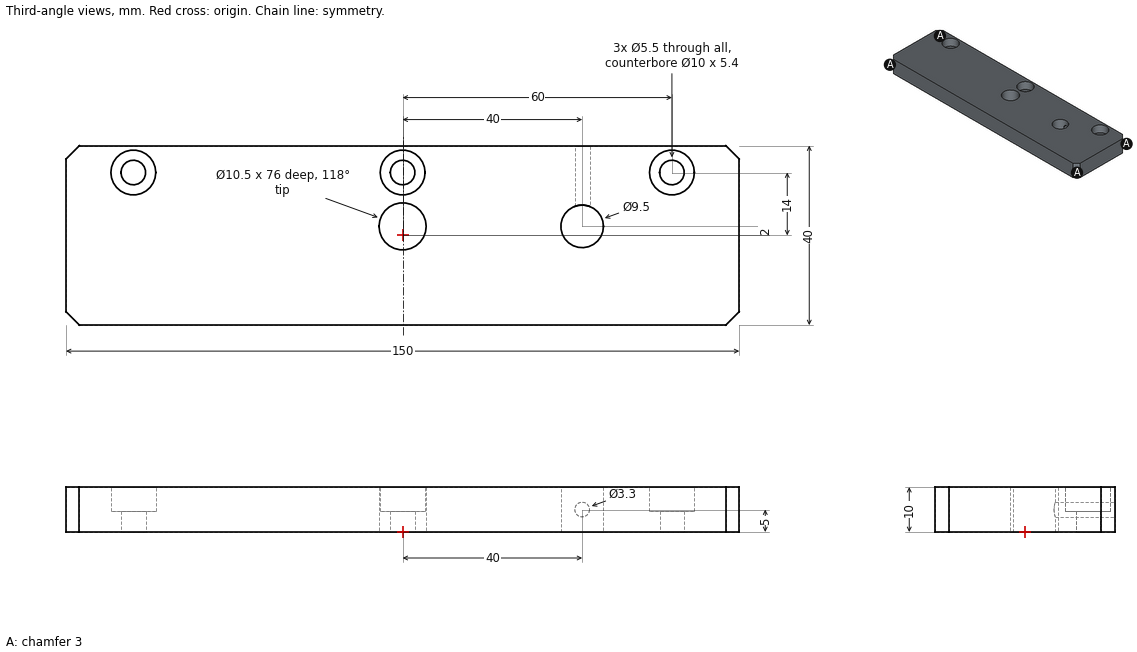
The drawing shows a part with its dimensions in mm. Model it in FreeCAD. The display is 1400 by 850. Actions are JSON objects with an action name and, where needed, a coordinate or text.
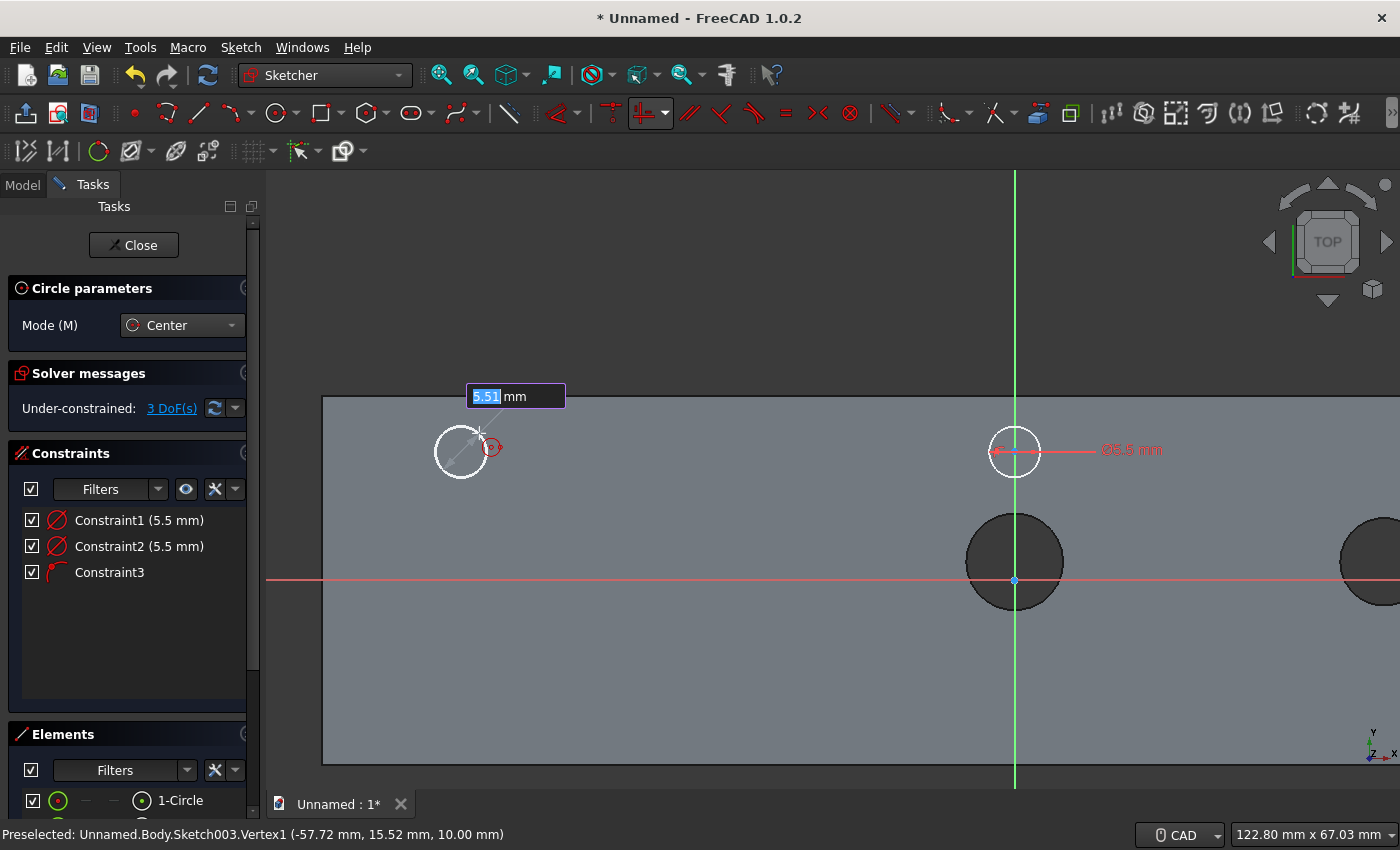
{"action": "type", "text": "5.5"}
{"action": "key", "text": "Return"}
{"action": "key", "text": "Escape"}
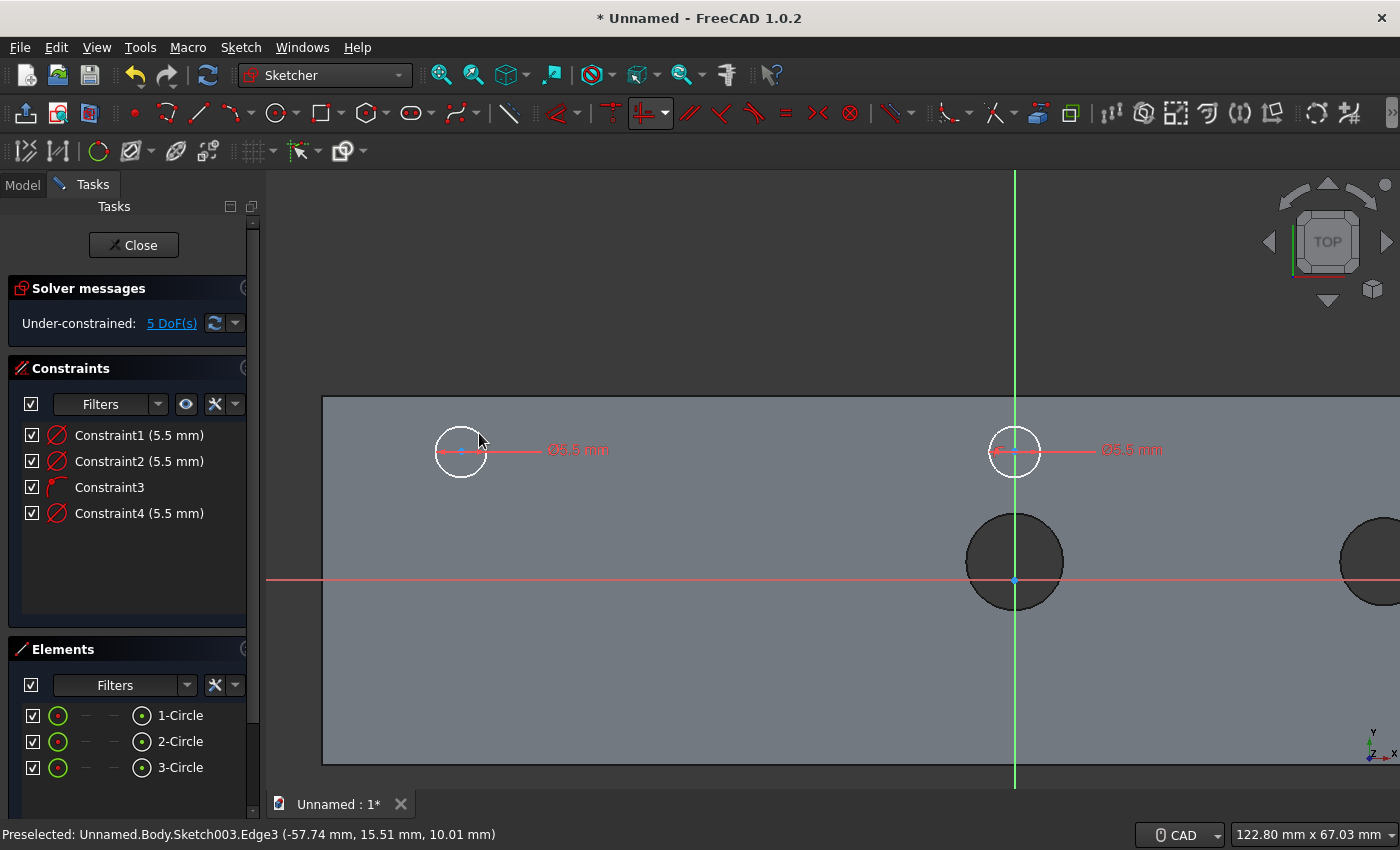
{"action": "scroll", "coordinate": [460, 451], "scroll_direction": "down", "scroll_amount": 3}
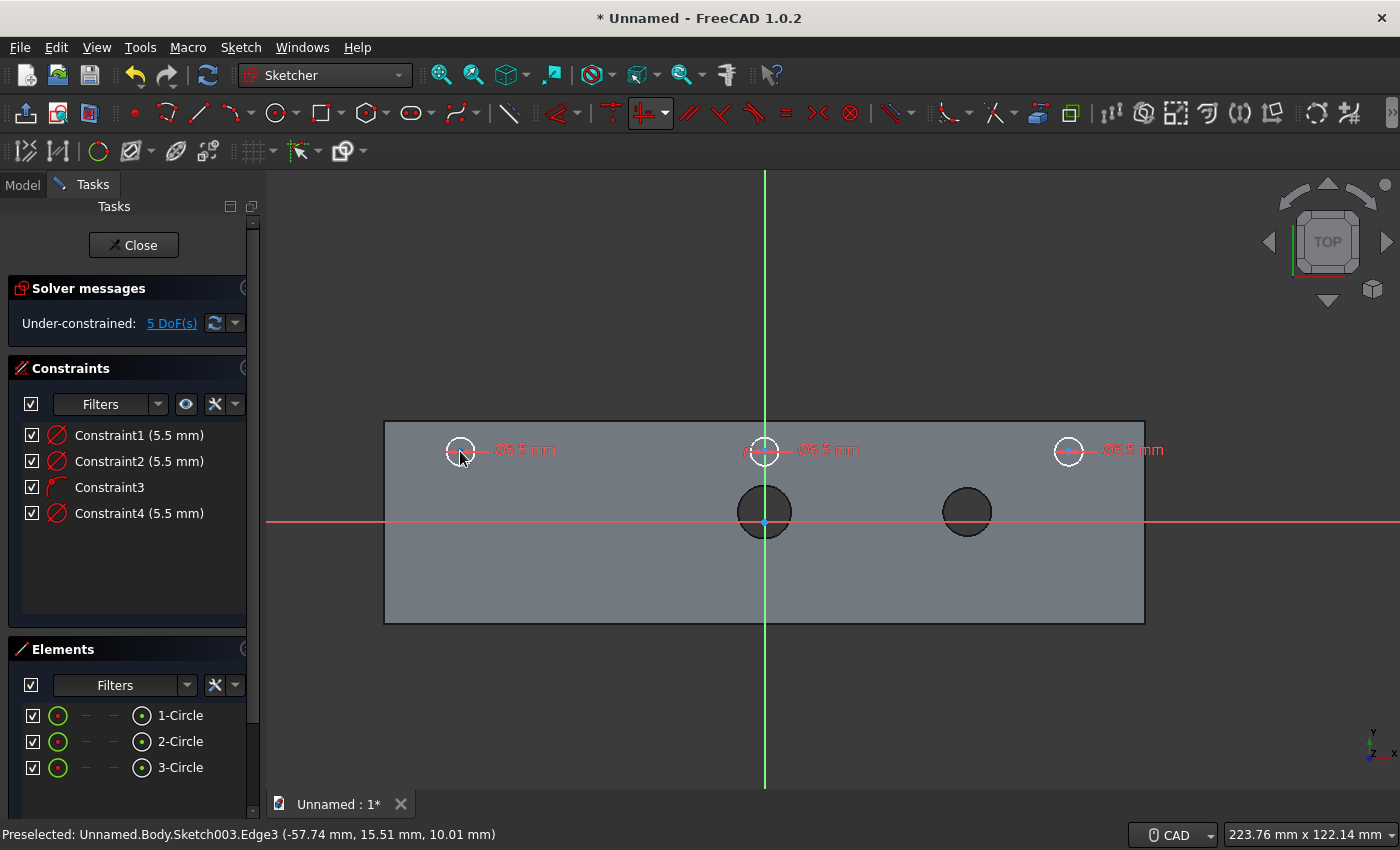
{"action": "left_click", "coordinate": [1069, 452]}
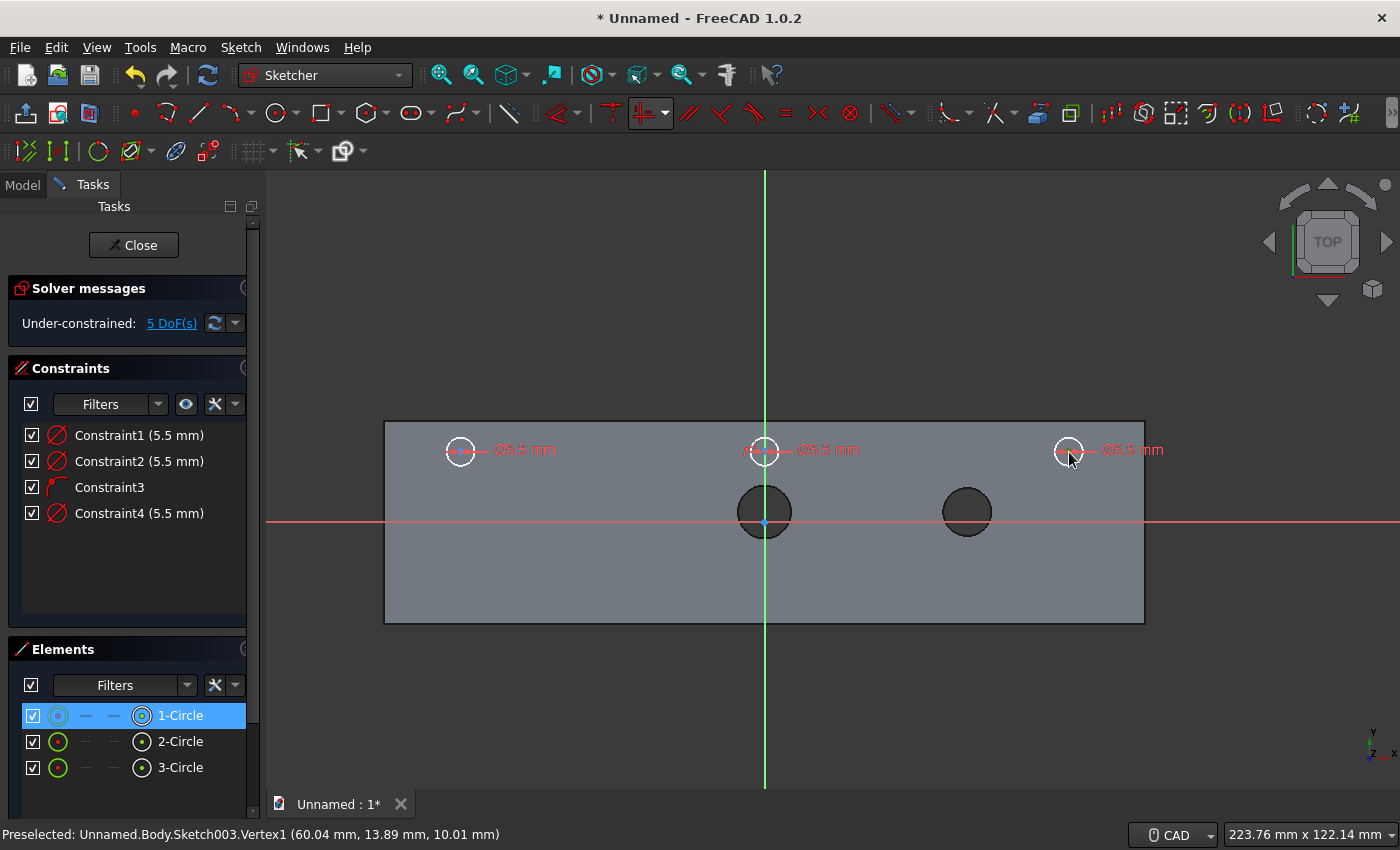
{"action": "left_click", "coordinate": [461, 452]}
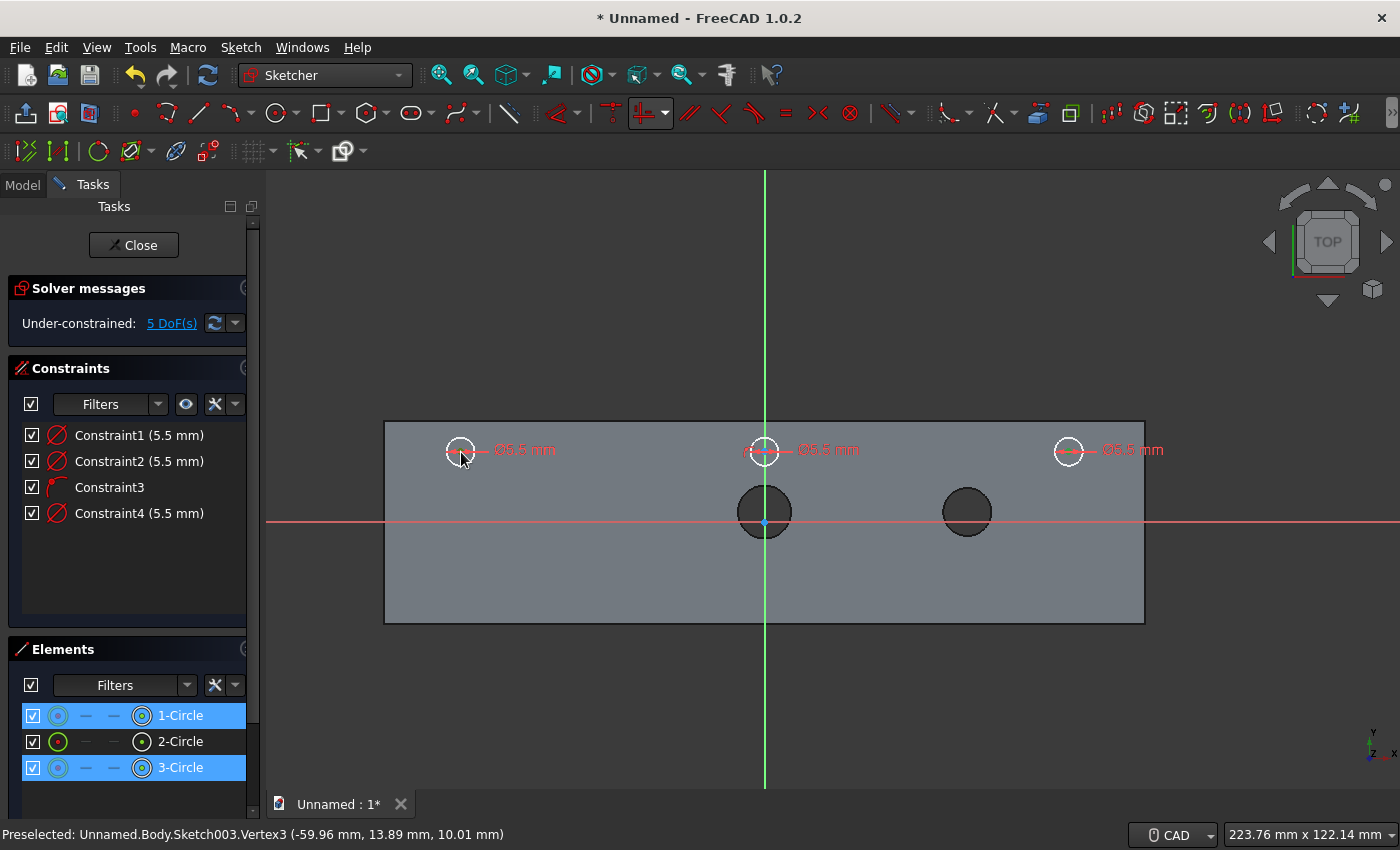
{"action": "left_click", "coordinate": [765, 721]}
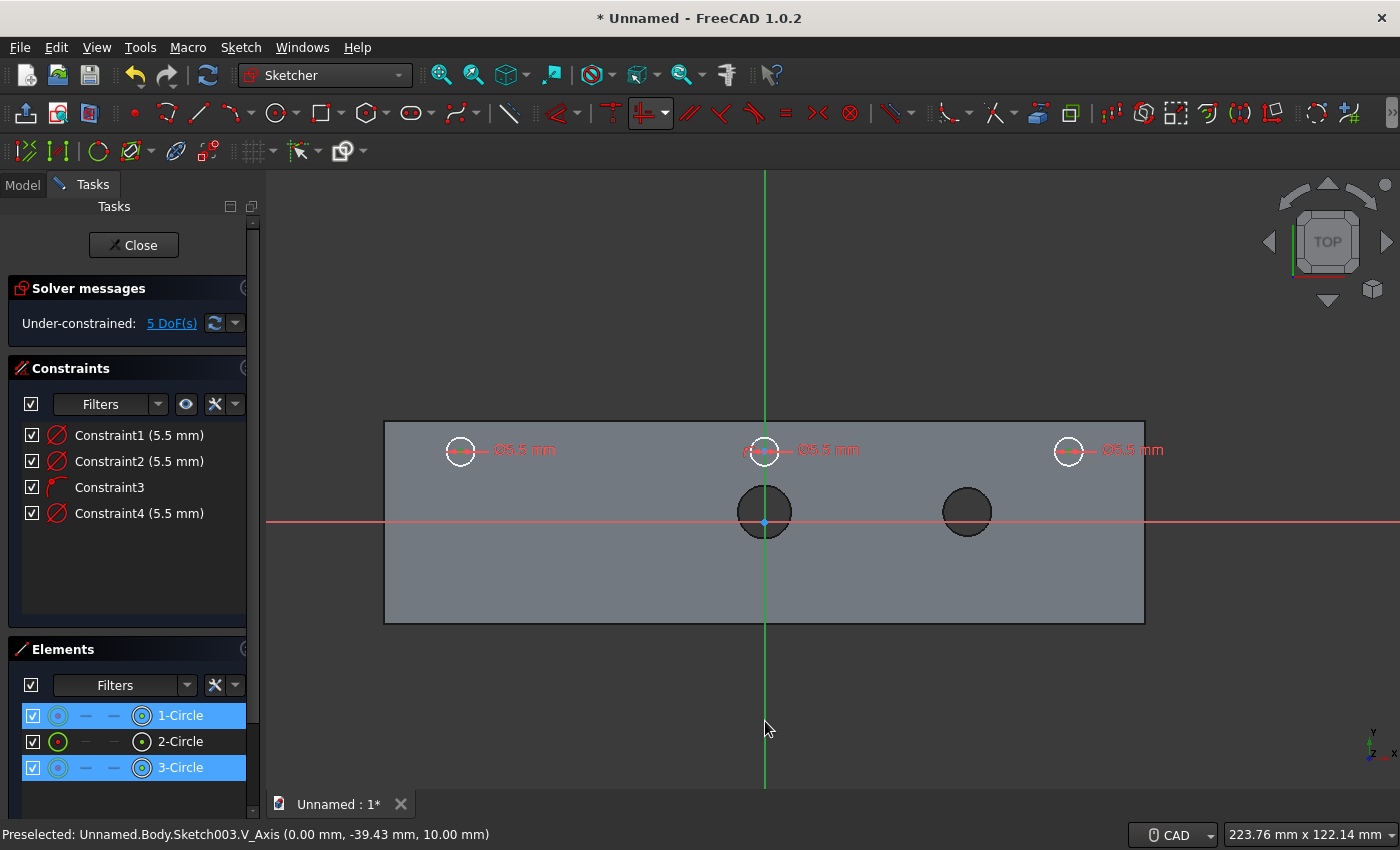
{"action": "key", "text": "s"}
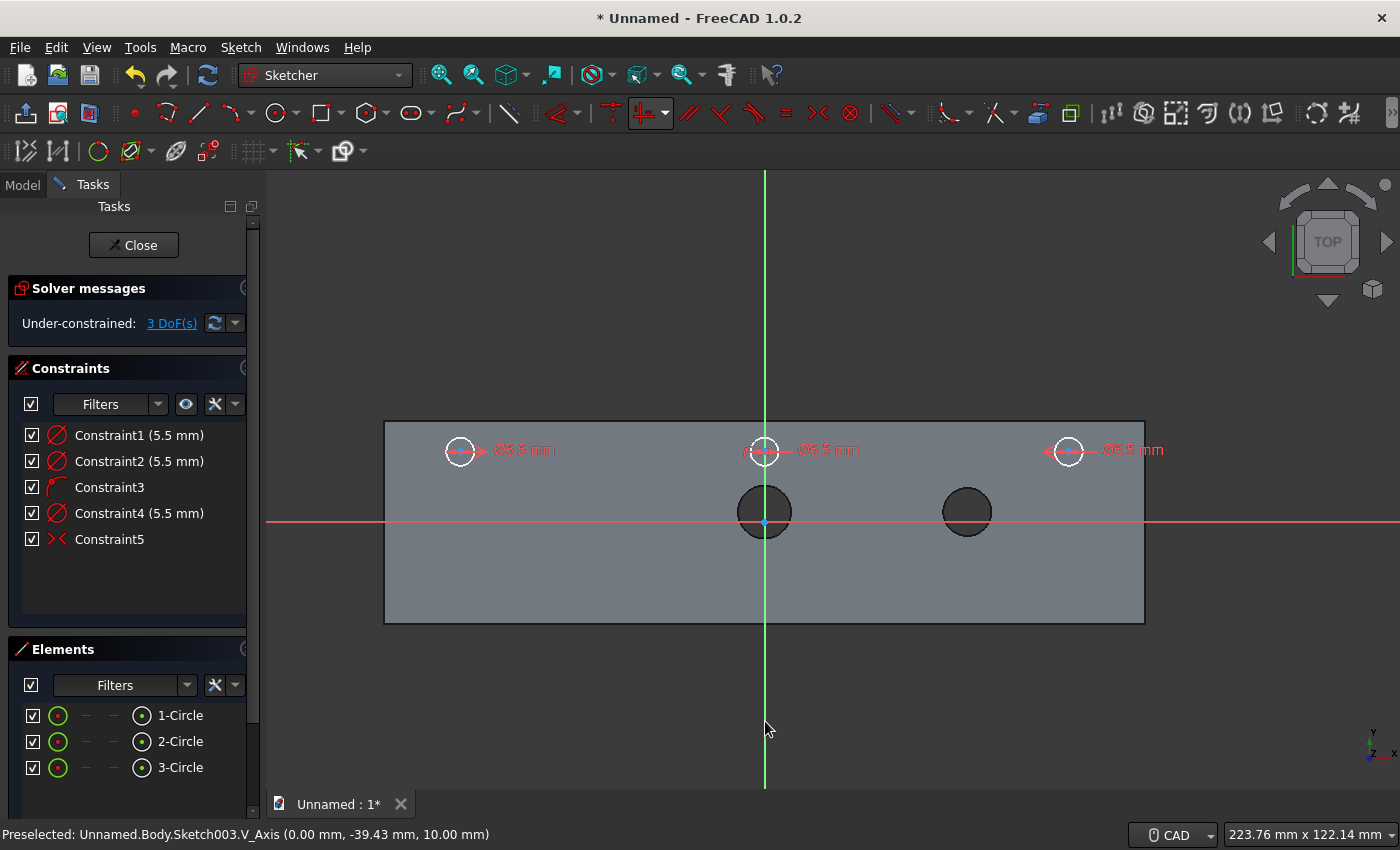
{"action": "left_click", "coordinate": [556, 114]}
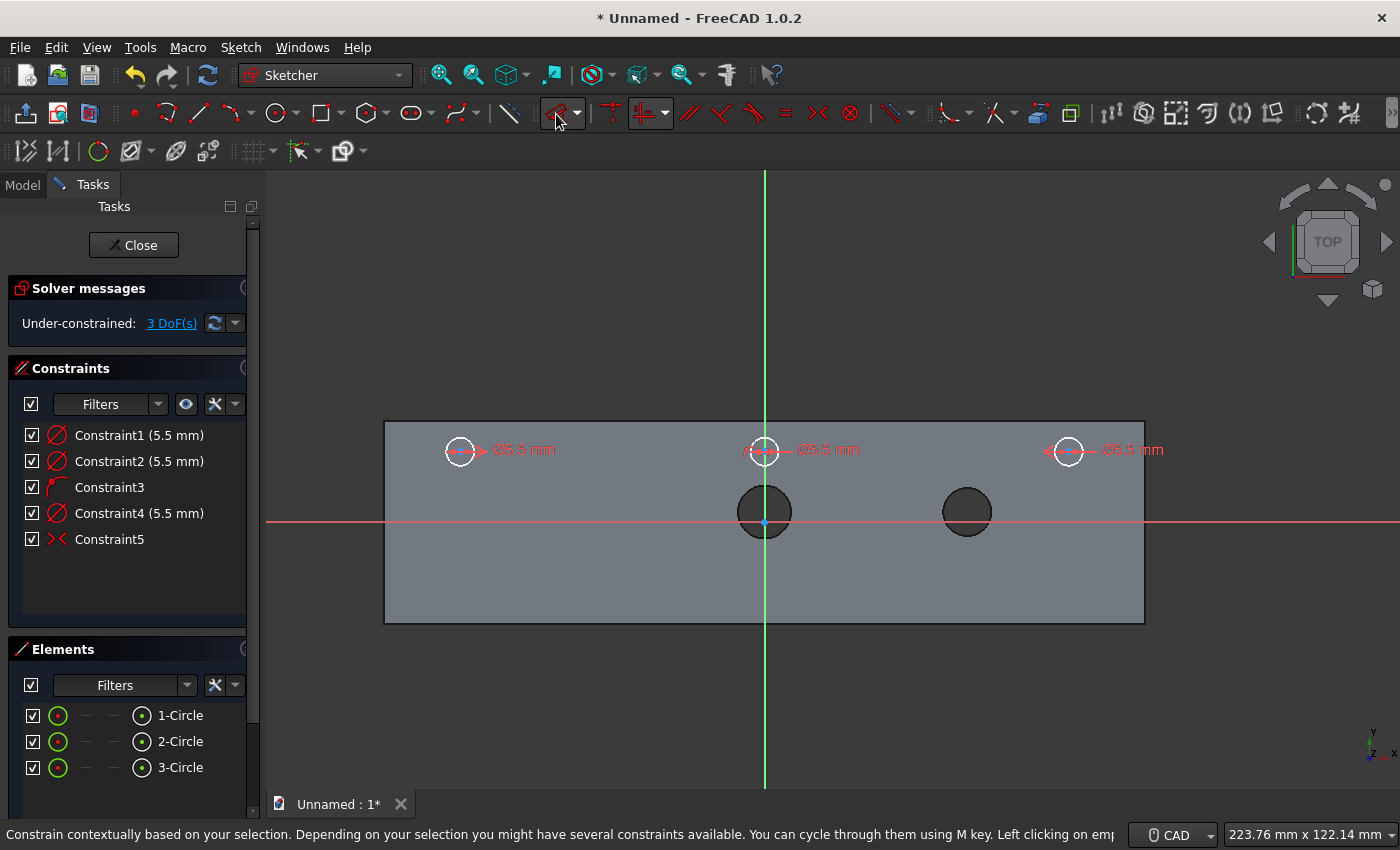
{"action": "left_click", "coordinate": [1069, 452]}
{"action": "left_click", "coordinate": [917, 556]}